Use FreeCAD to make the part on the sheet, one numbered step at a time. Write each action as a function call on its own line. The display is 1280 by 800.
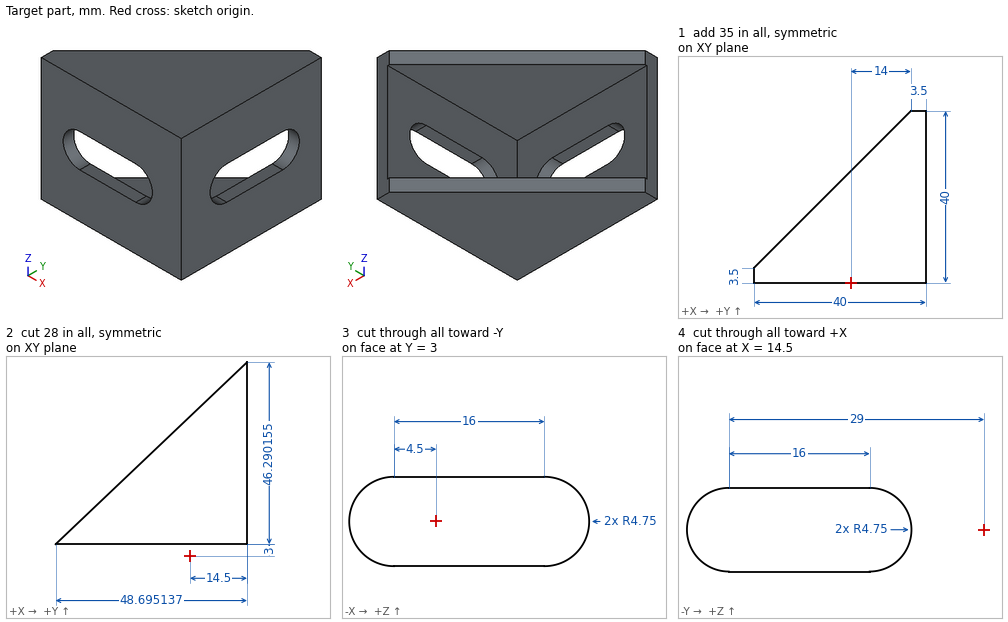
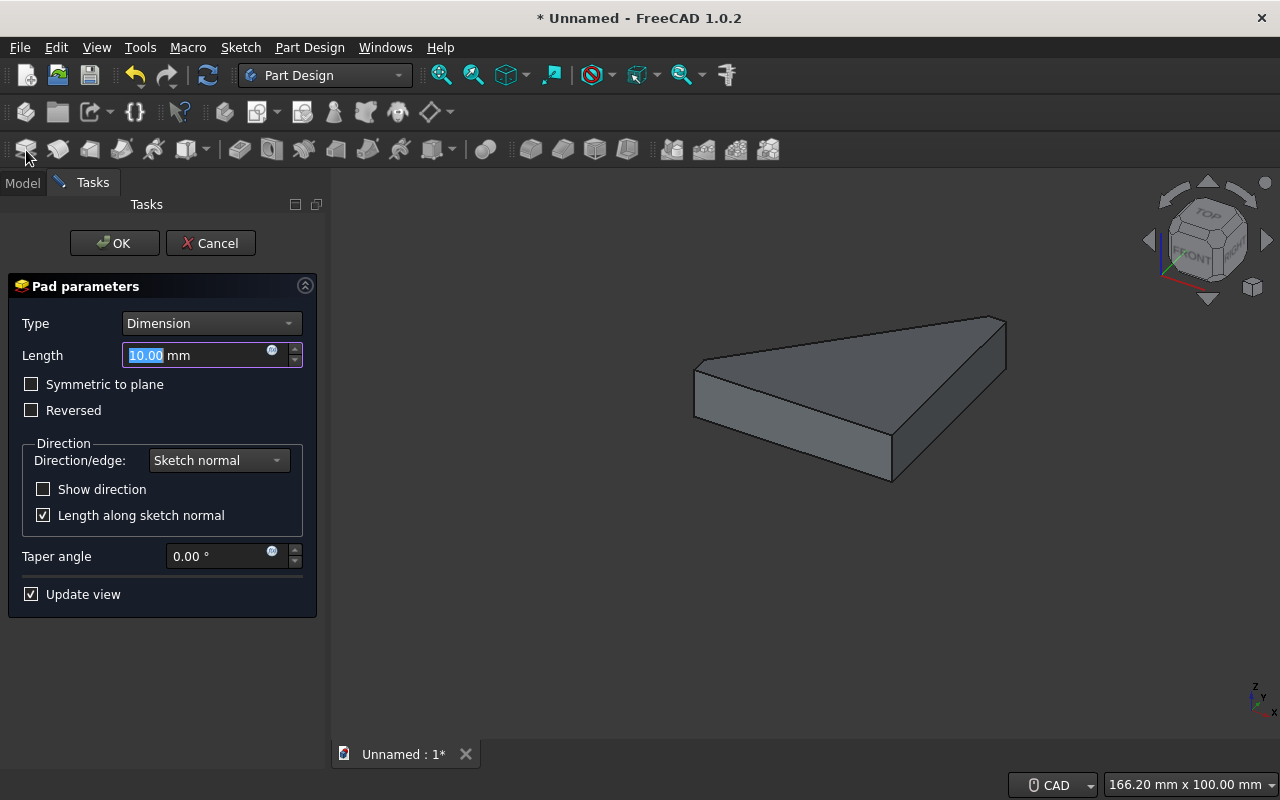
text(35)
key(Tab)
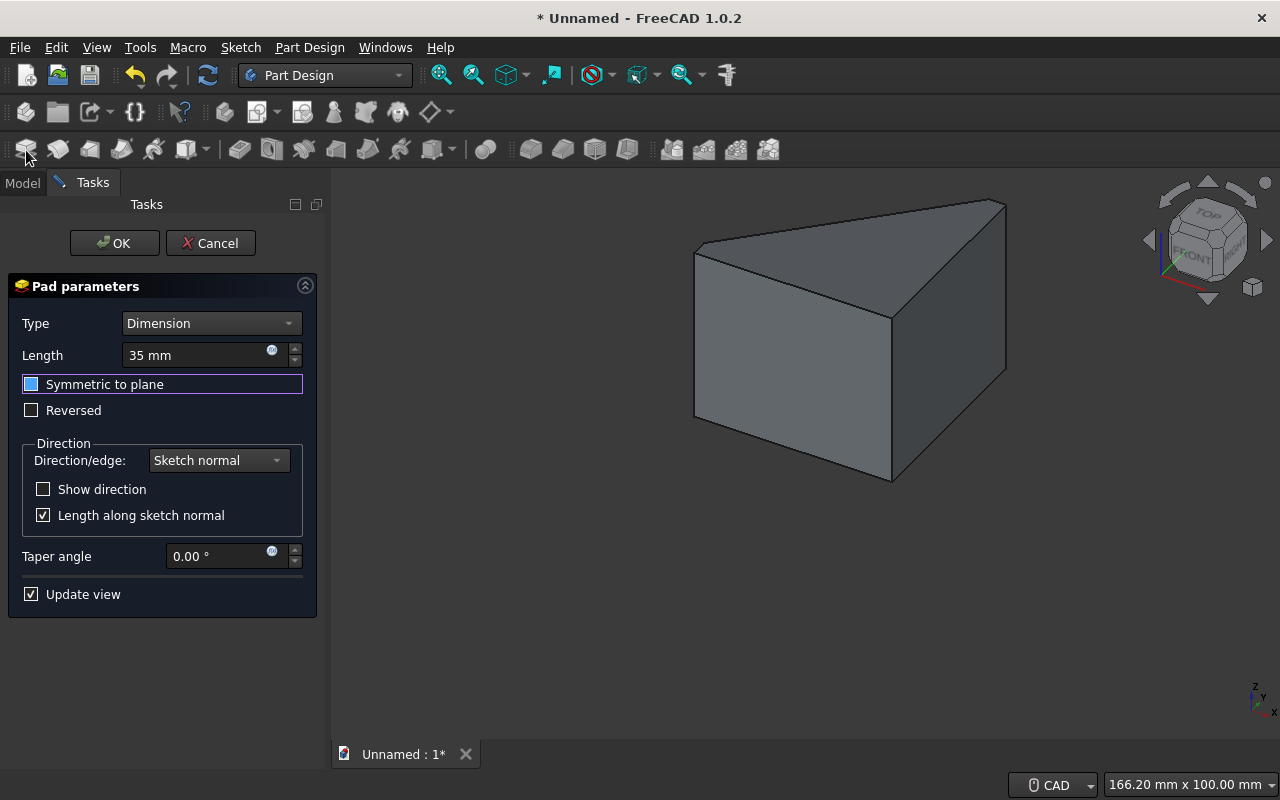
click(30, 384)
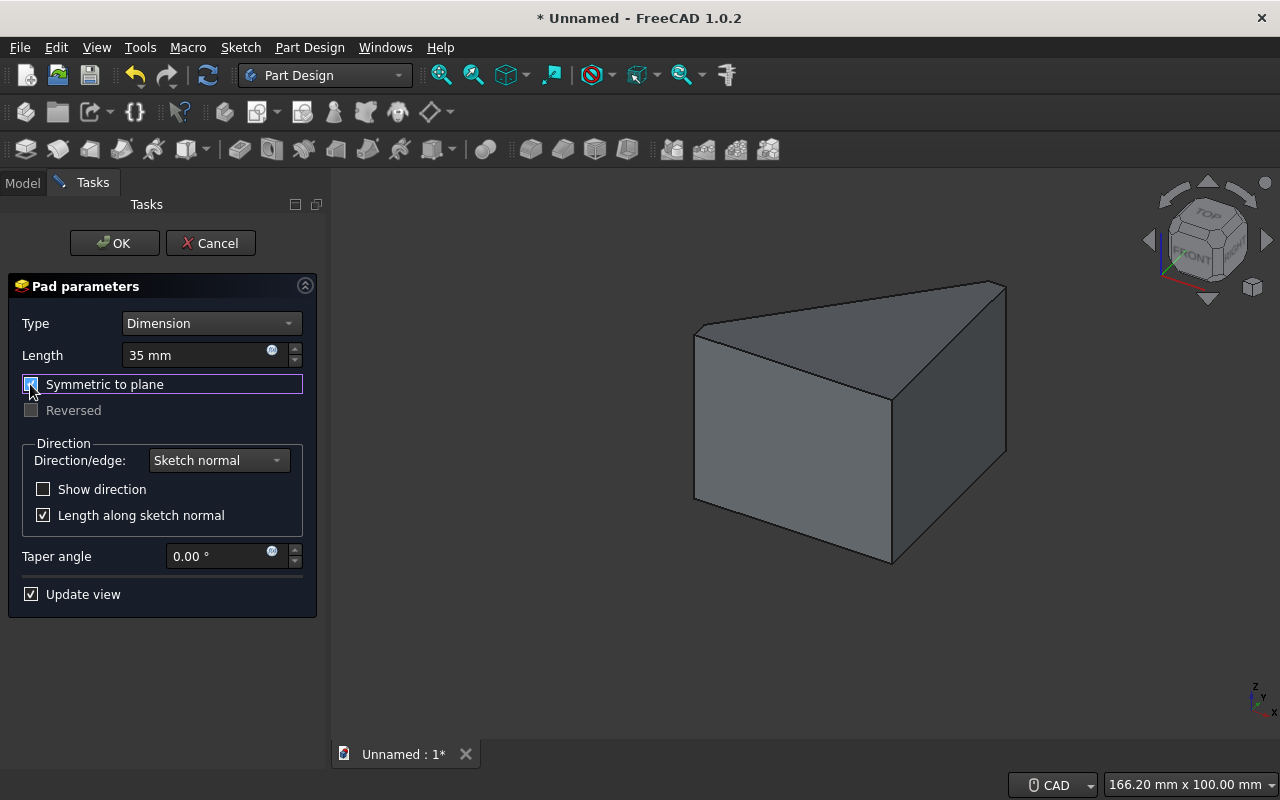
click(115, 243)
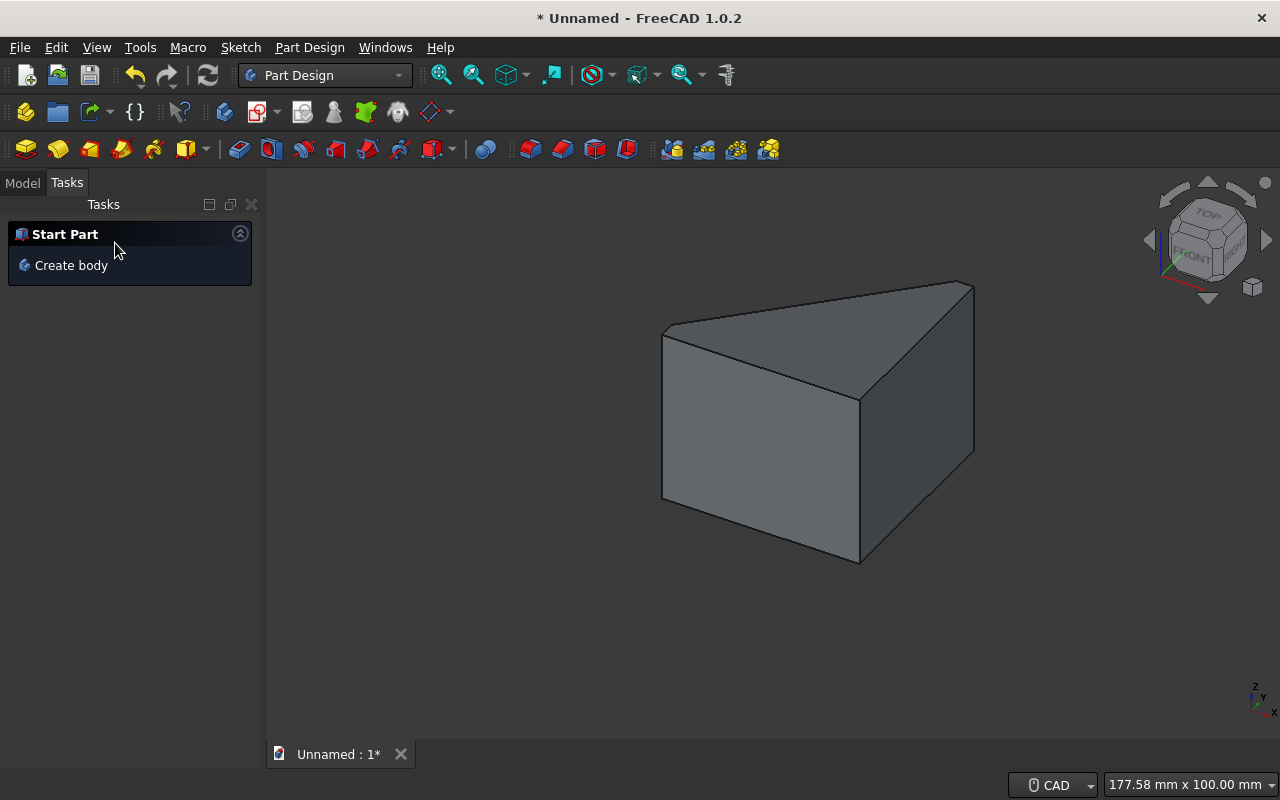
click(258, 112)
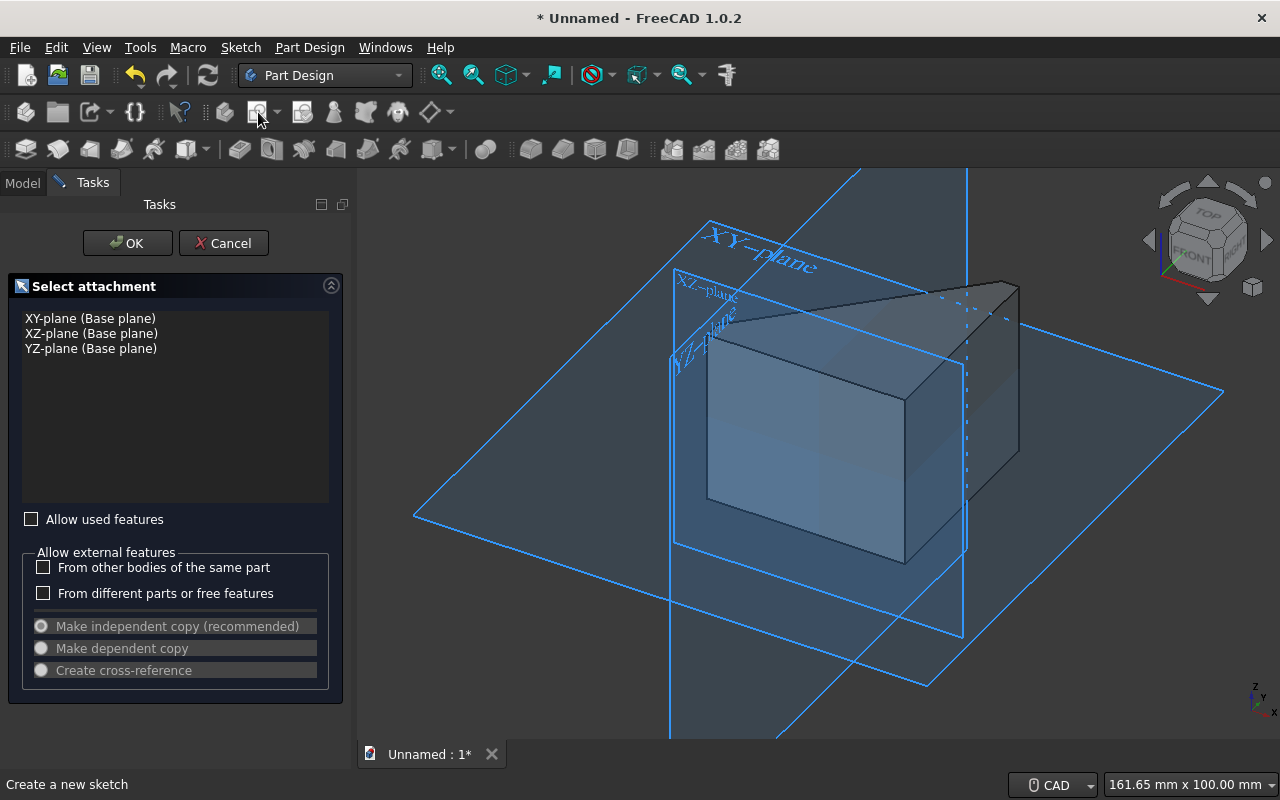
click(82, 318)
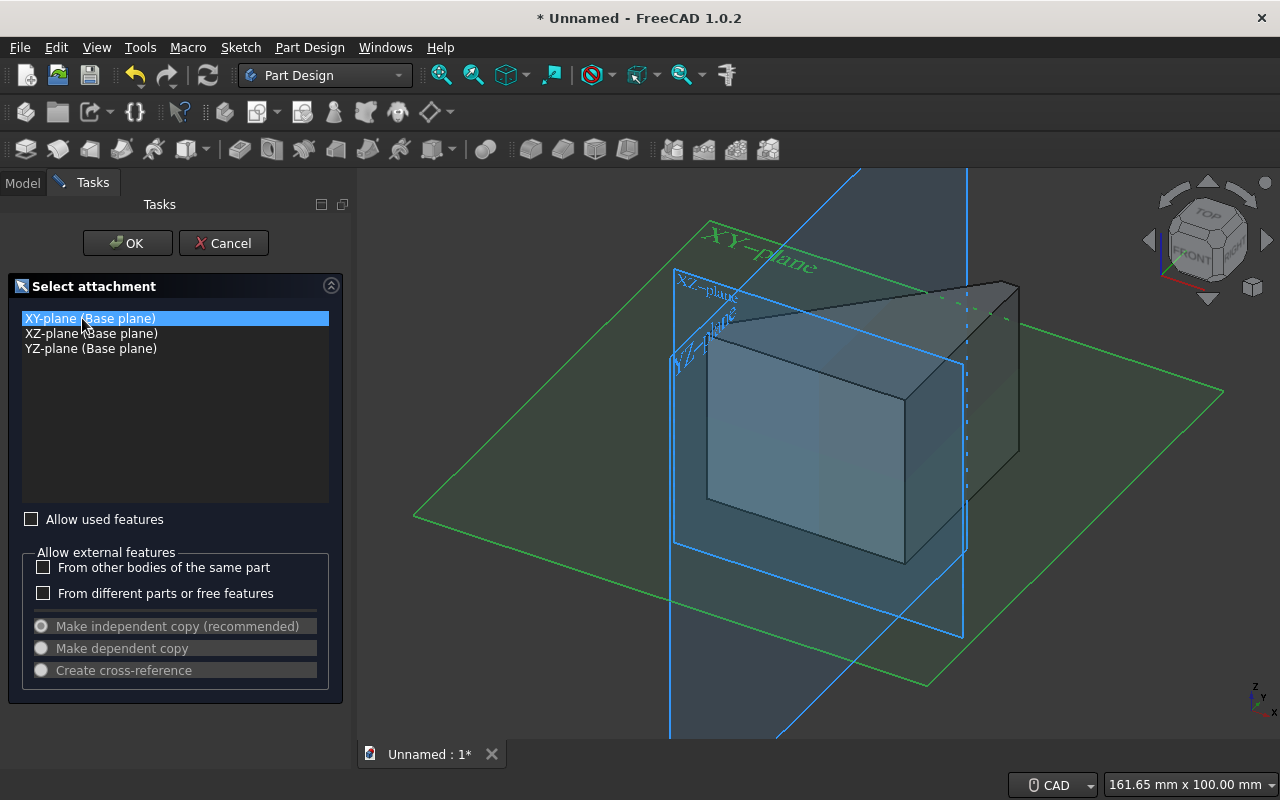
click(128, 243)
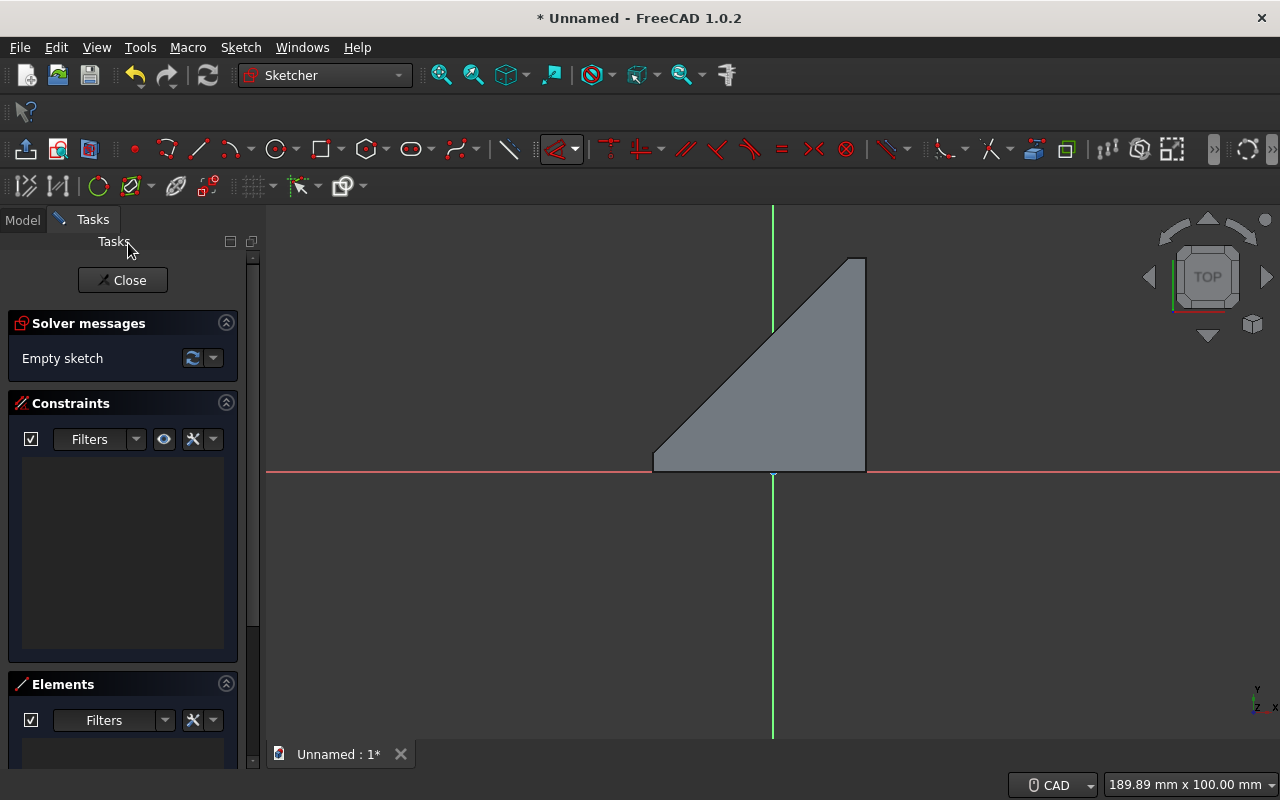
click(90, 150)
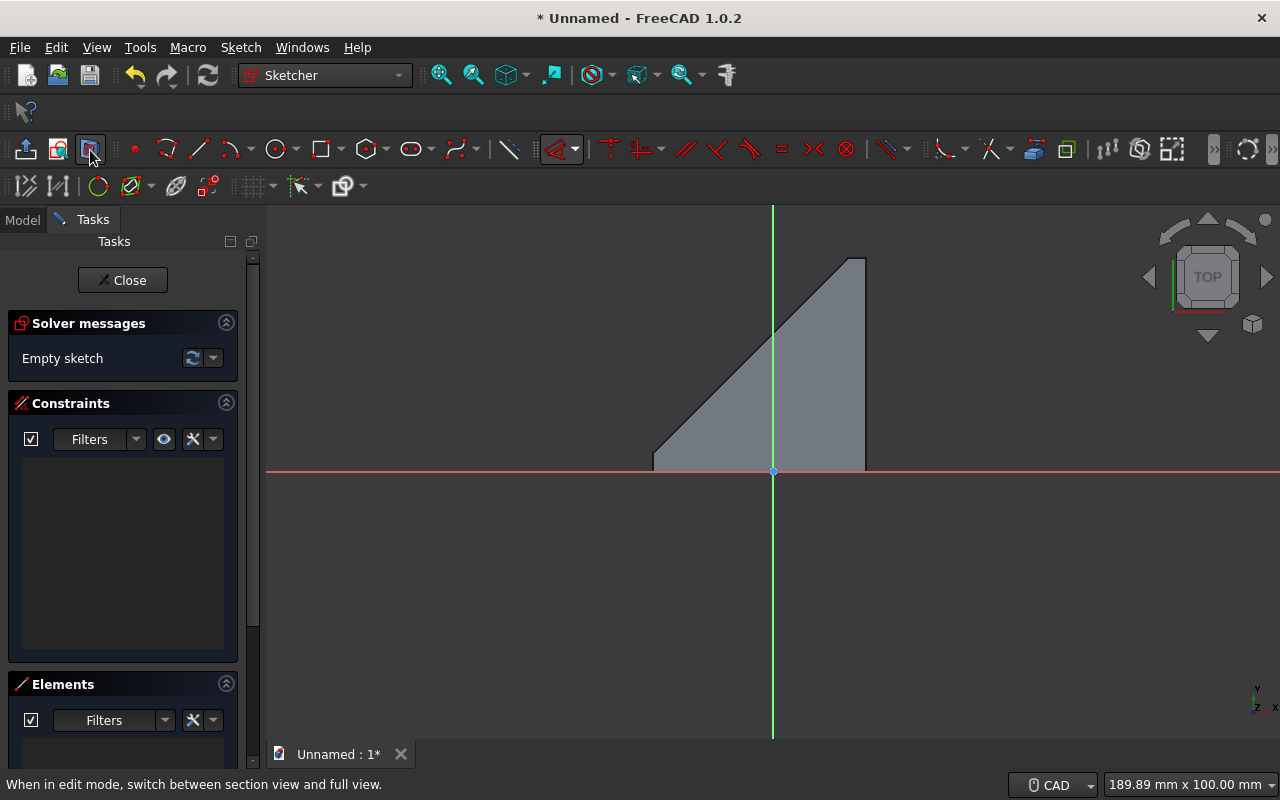
scroll(633, 711, down, 1)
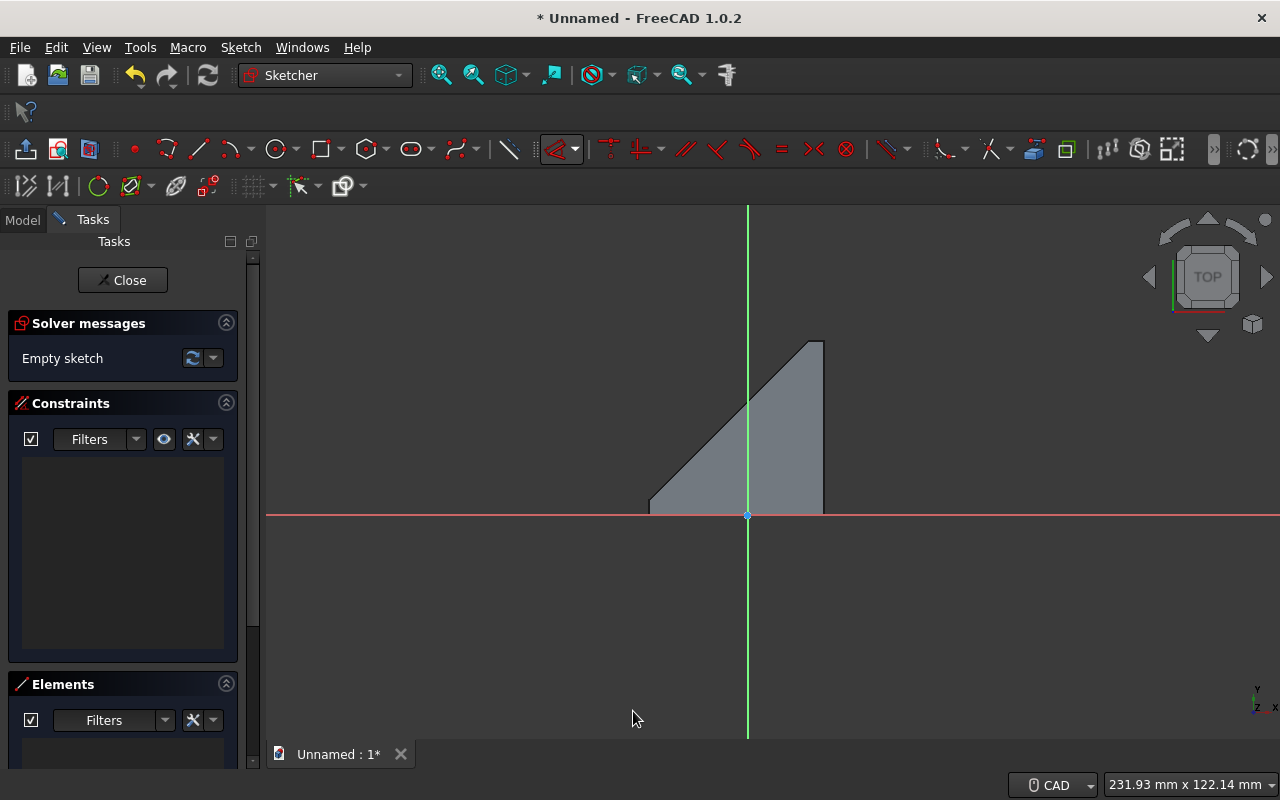
scroll(705, 277, up, 2)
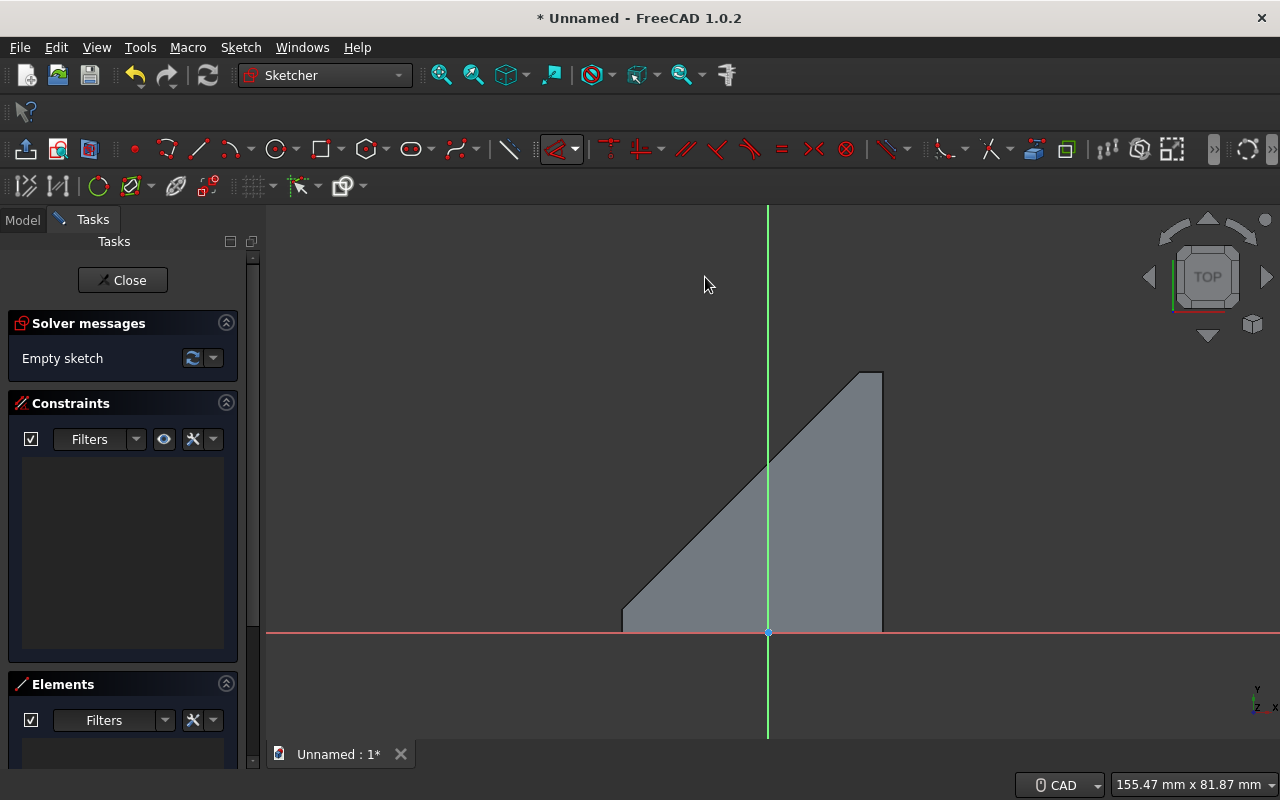
click(168, 150)